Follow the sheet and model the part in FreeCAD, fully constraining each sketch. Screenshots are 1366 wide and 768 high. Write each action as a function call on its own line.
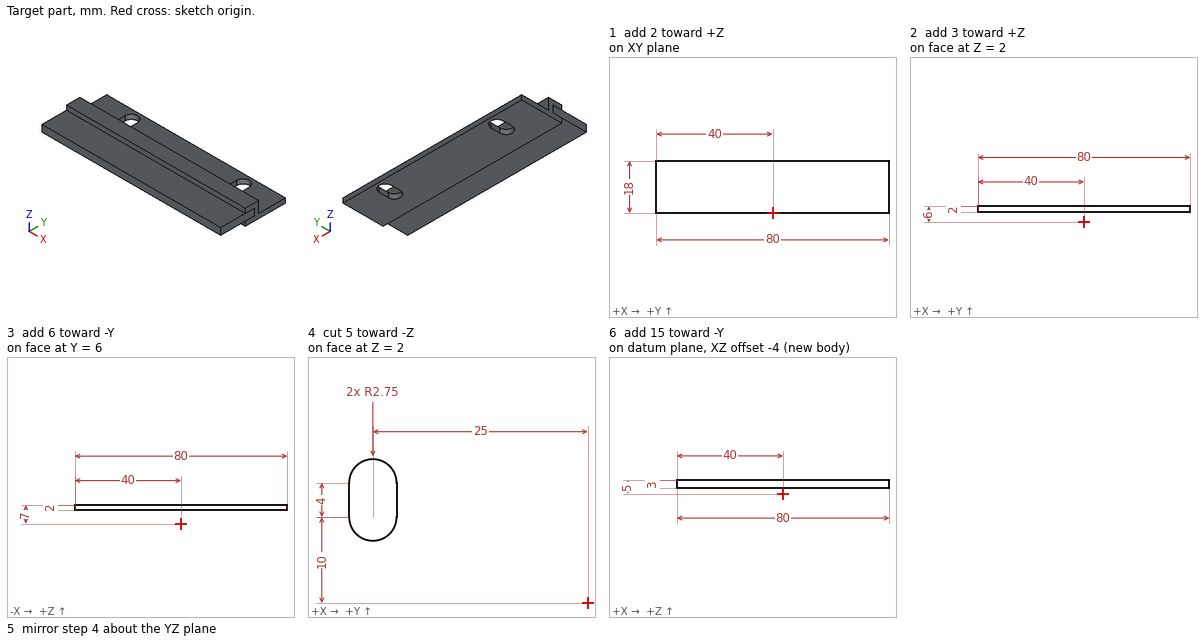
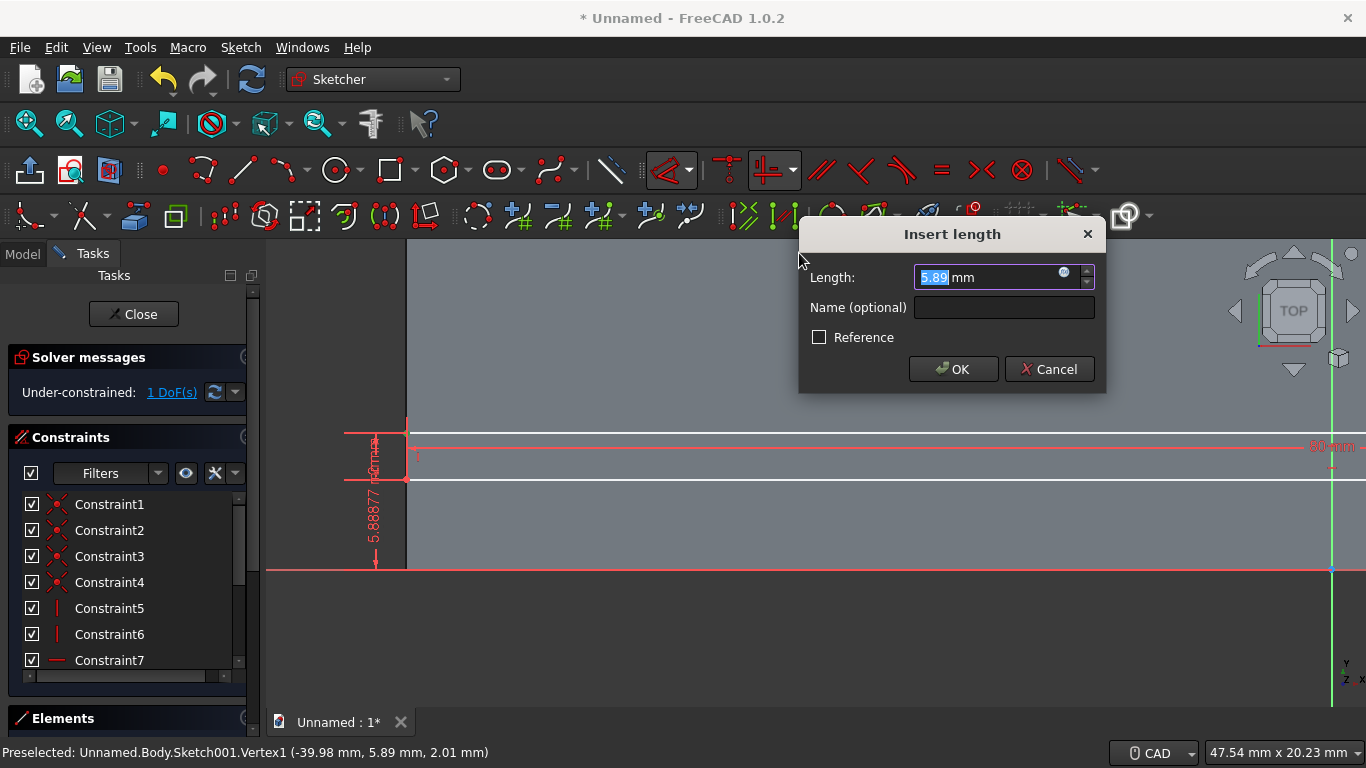
text(6)
key(Return)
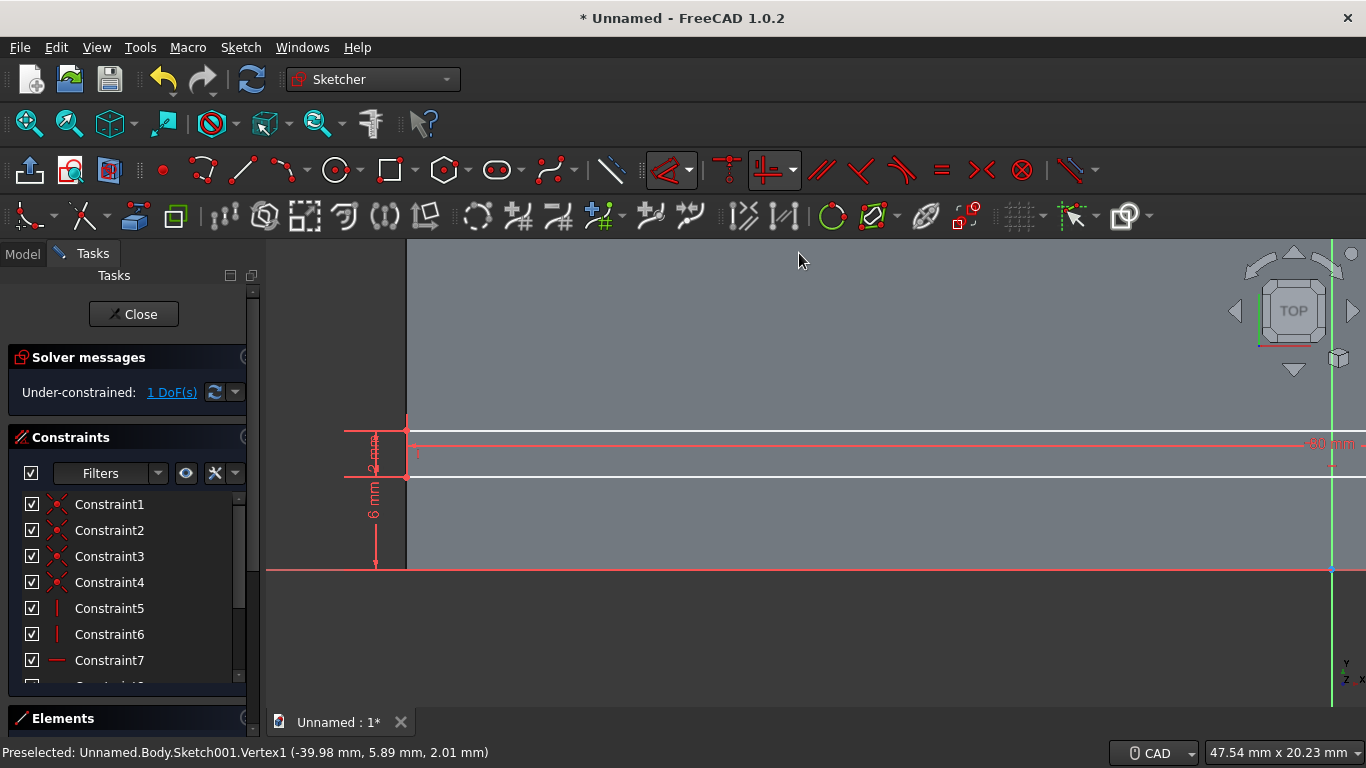
click(407, 431)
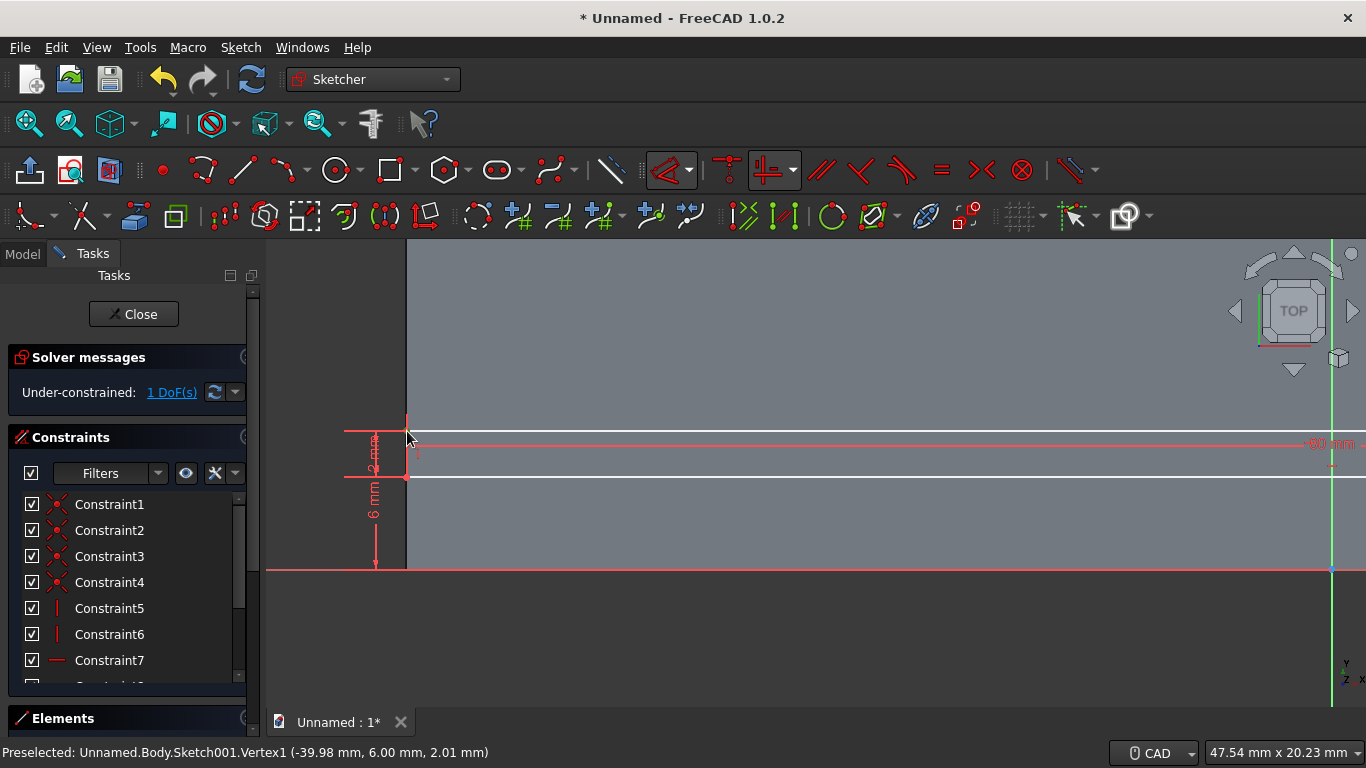
click(692, 170)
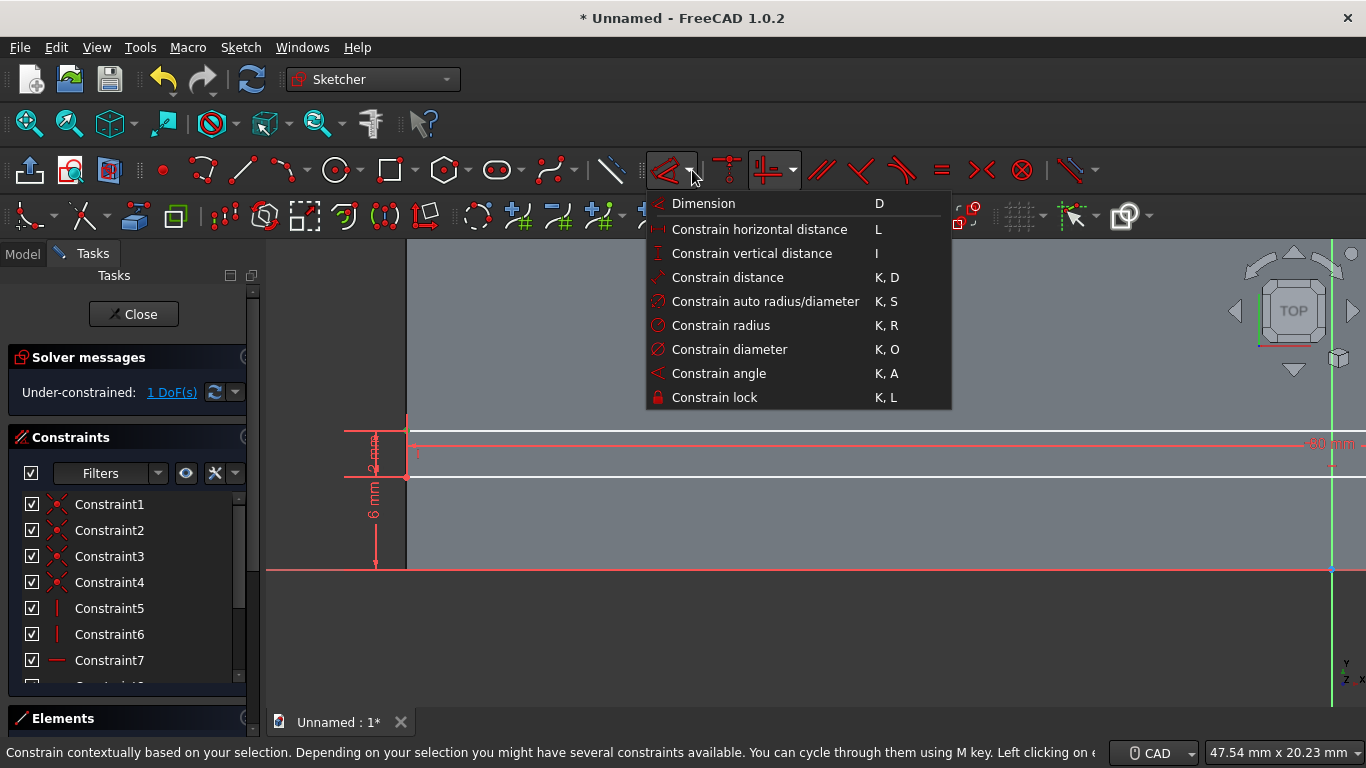
click(799, 229)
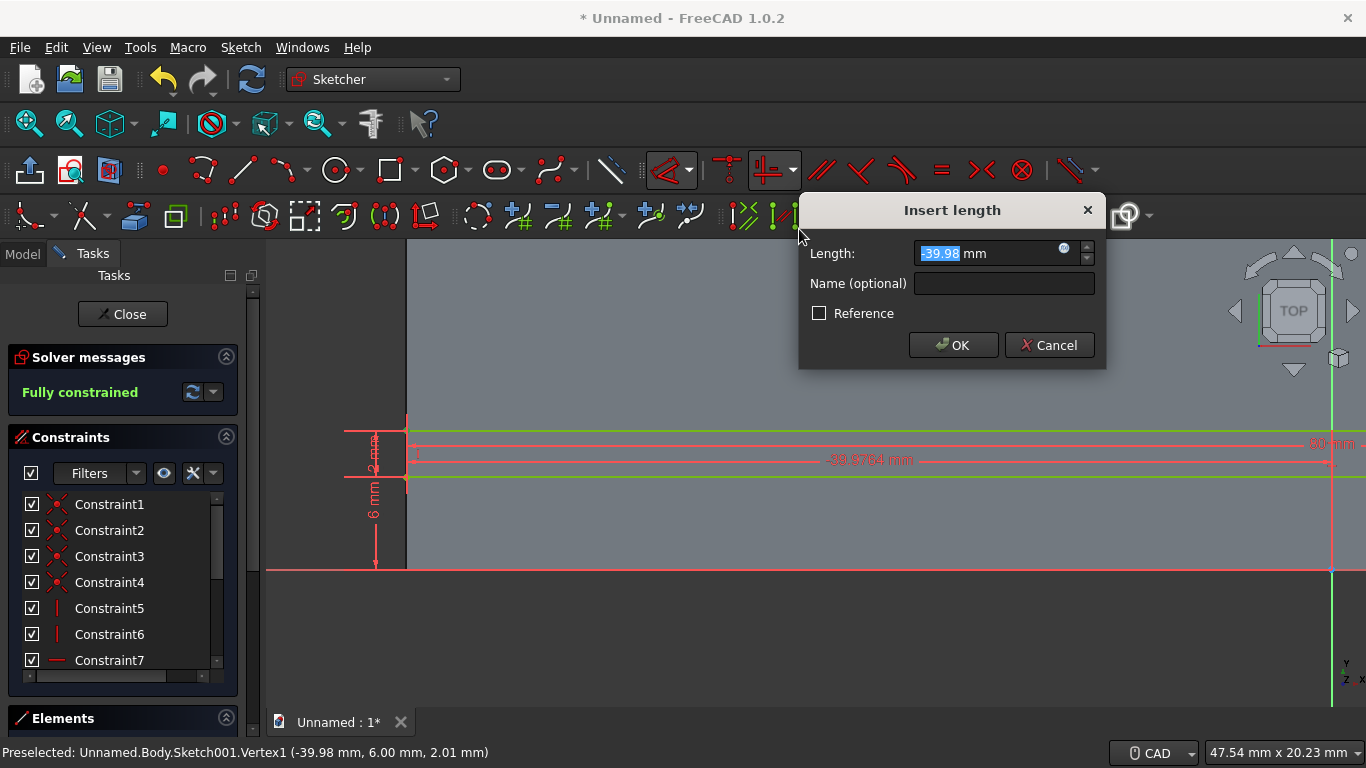
text(-40)
key(Return)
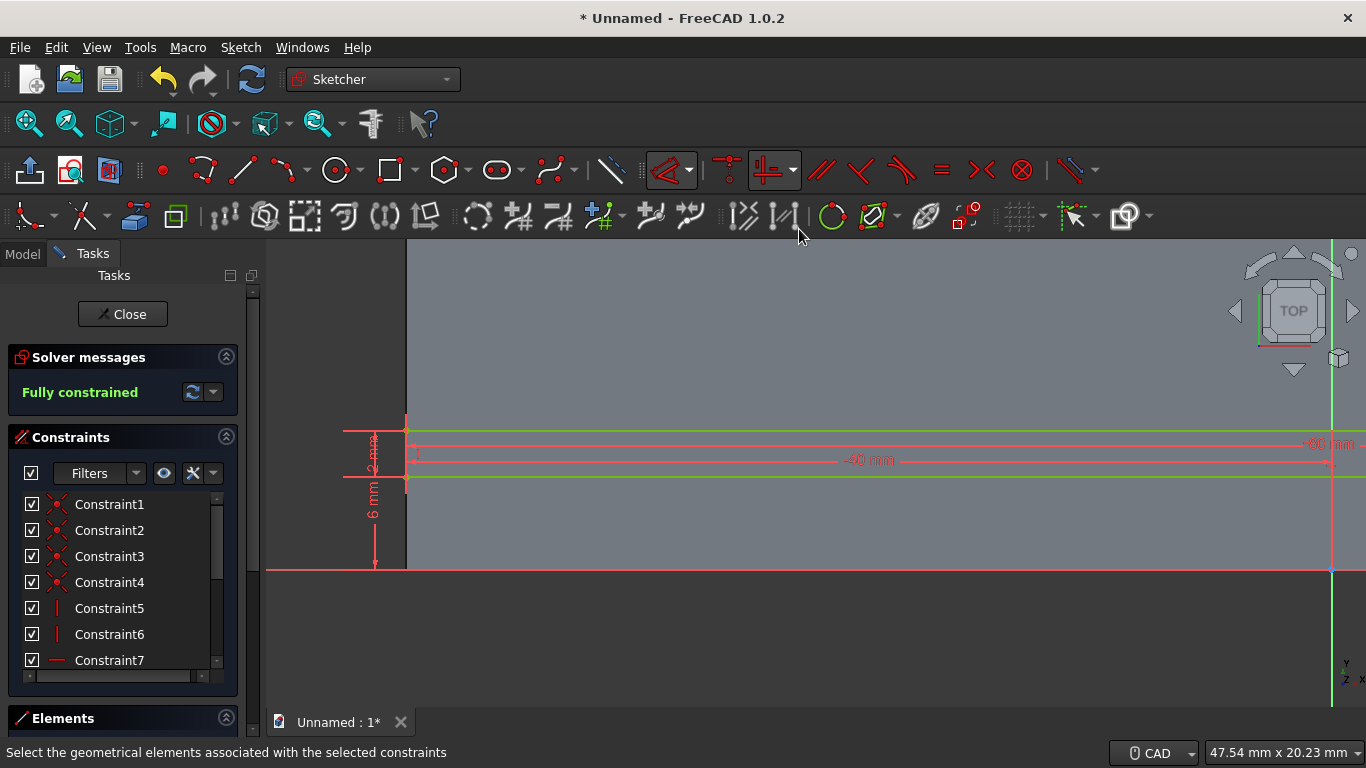
click(123, 314)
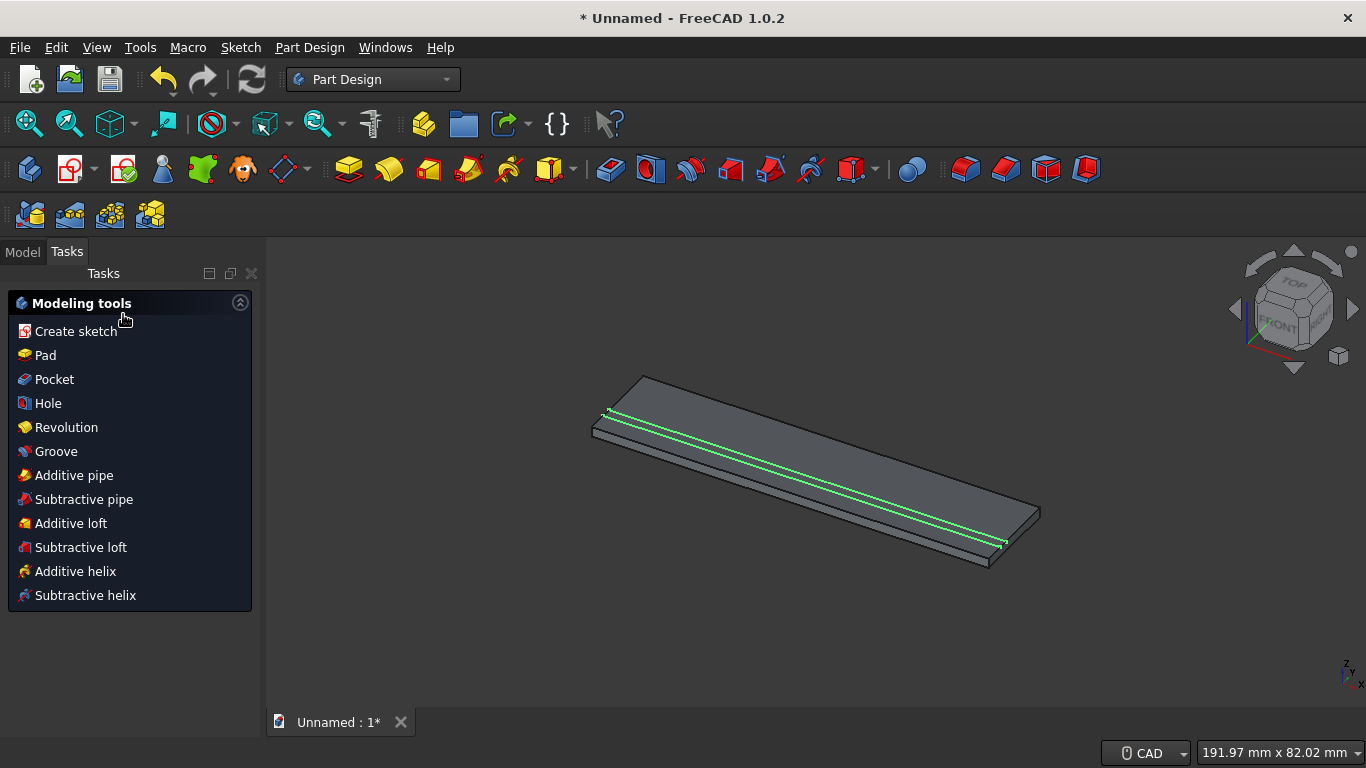
click(350, 170)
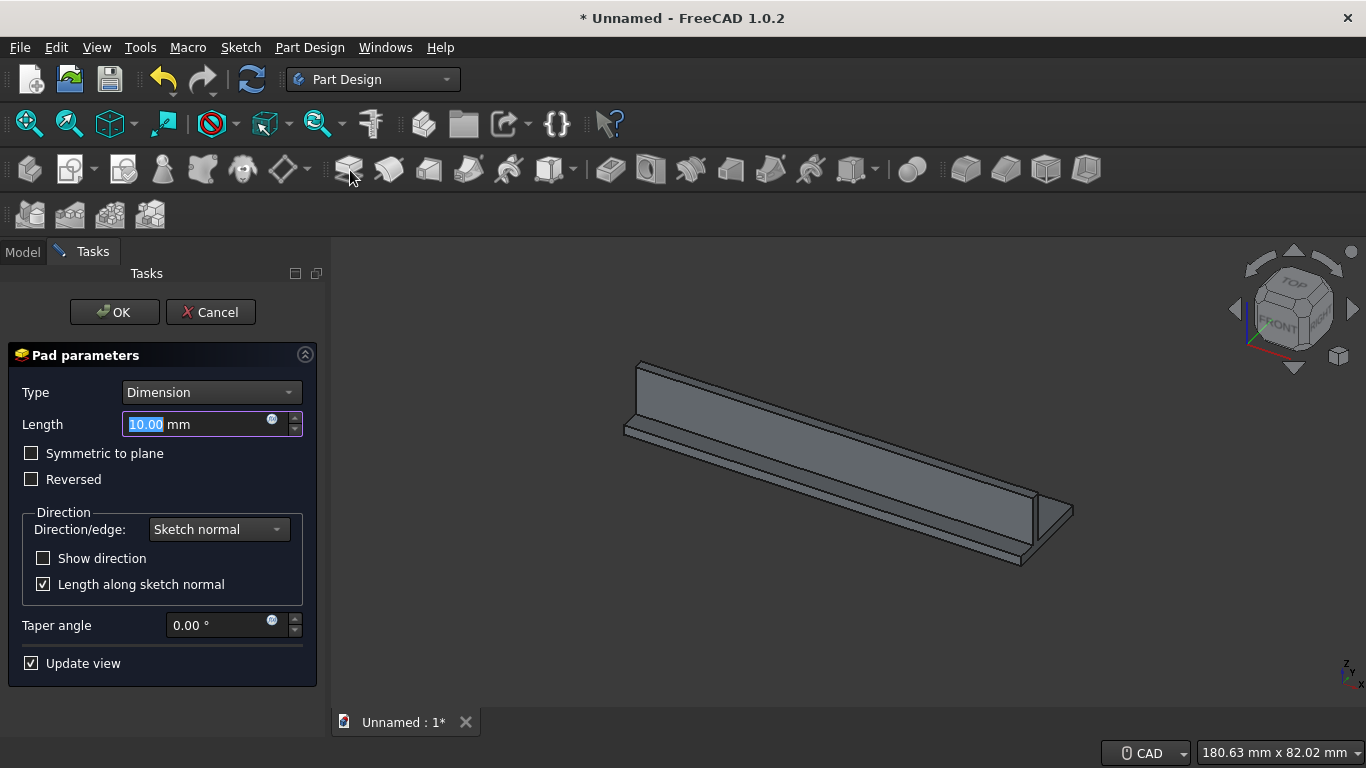
text(3)
key(Tab)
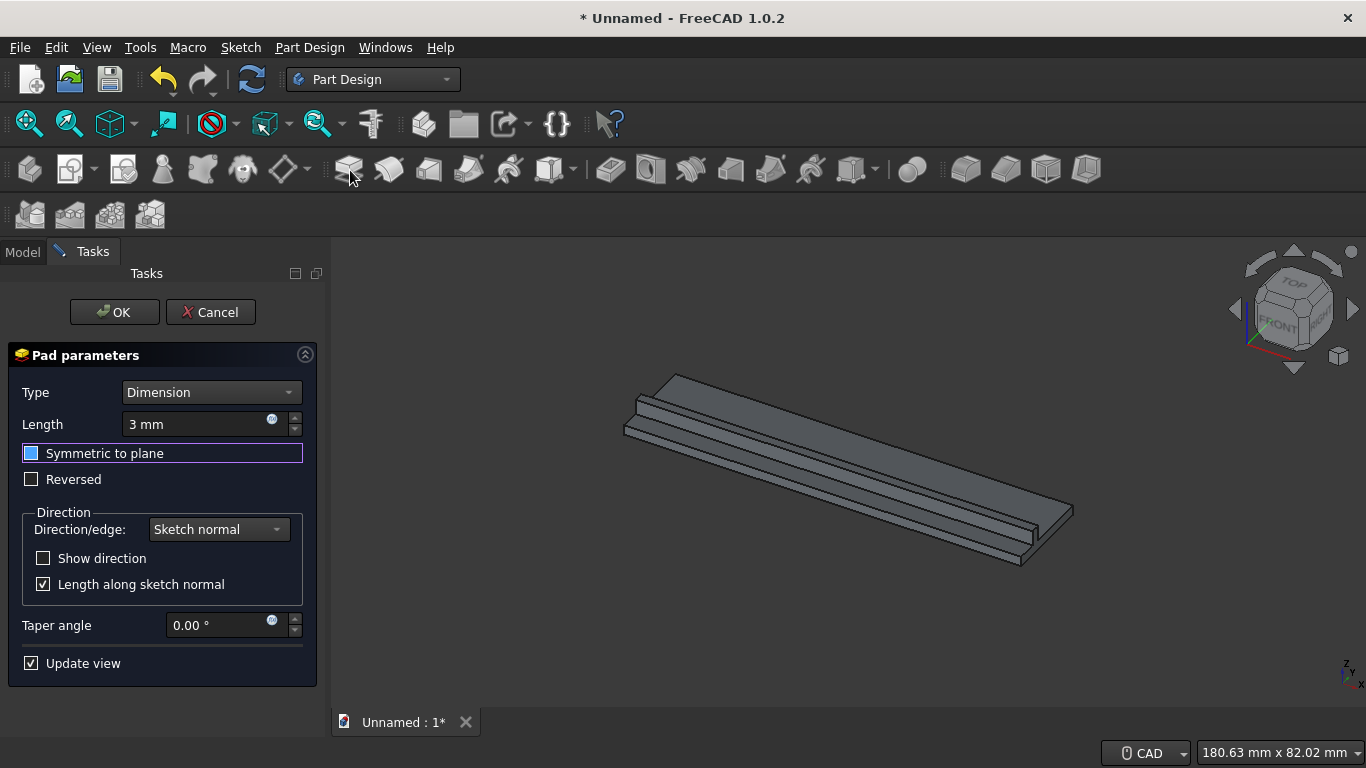
click(115, 312)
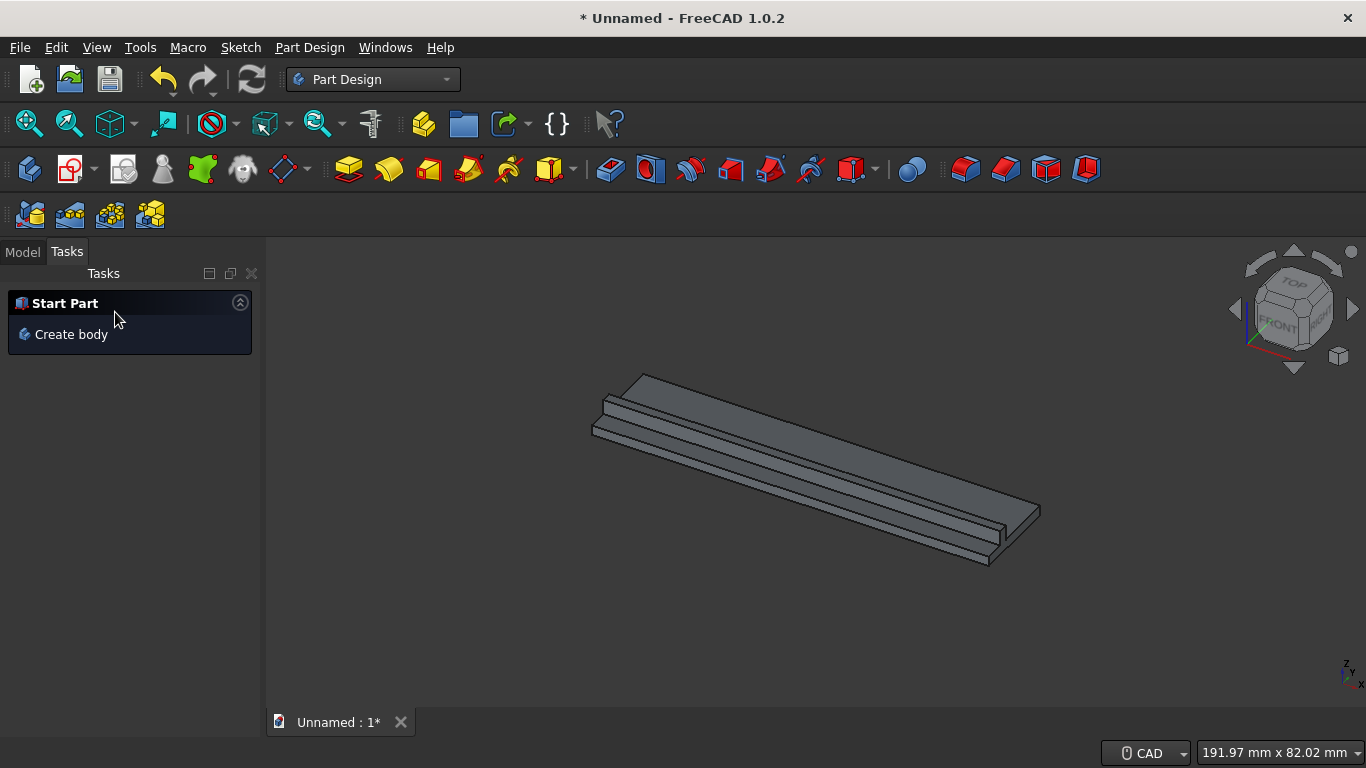
click(30, 124)